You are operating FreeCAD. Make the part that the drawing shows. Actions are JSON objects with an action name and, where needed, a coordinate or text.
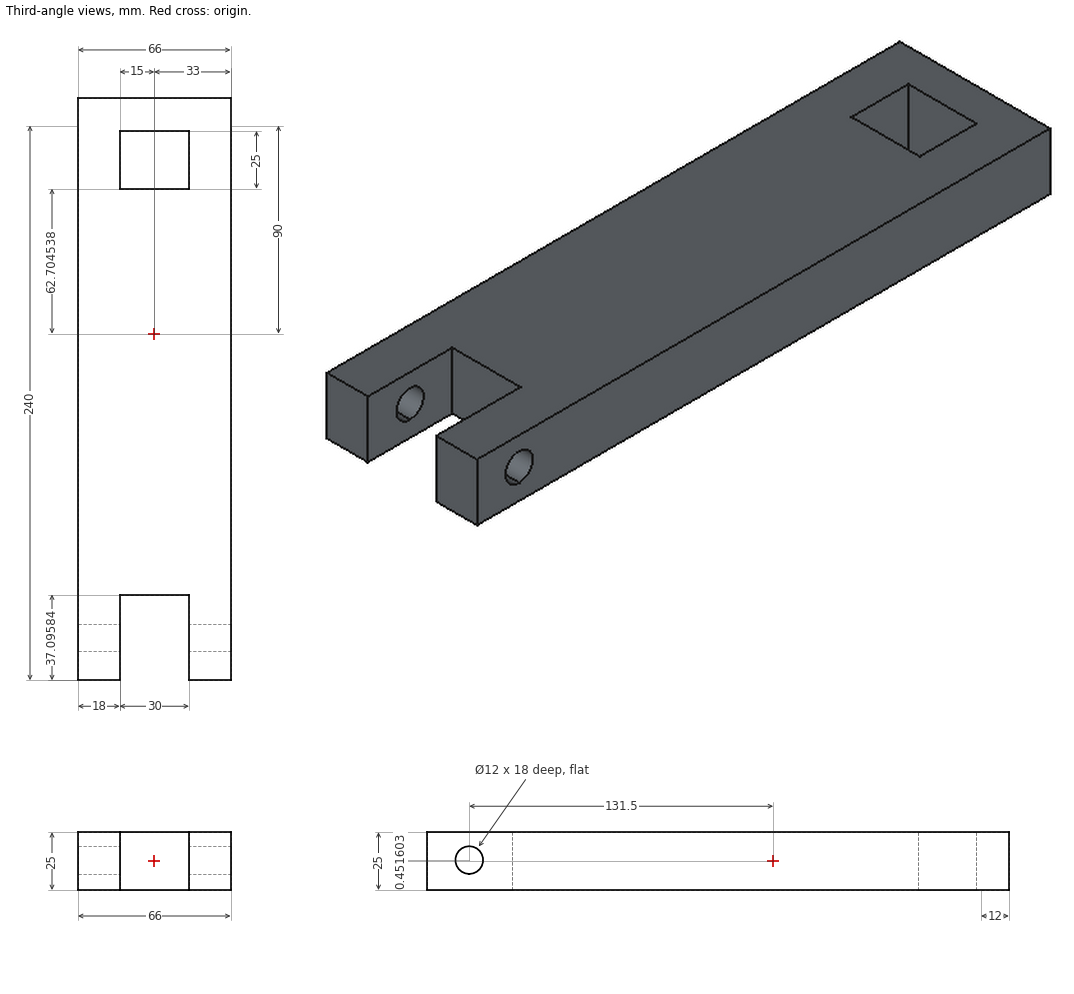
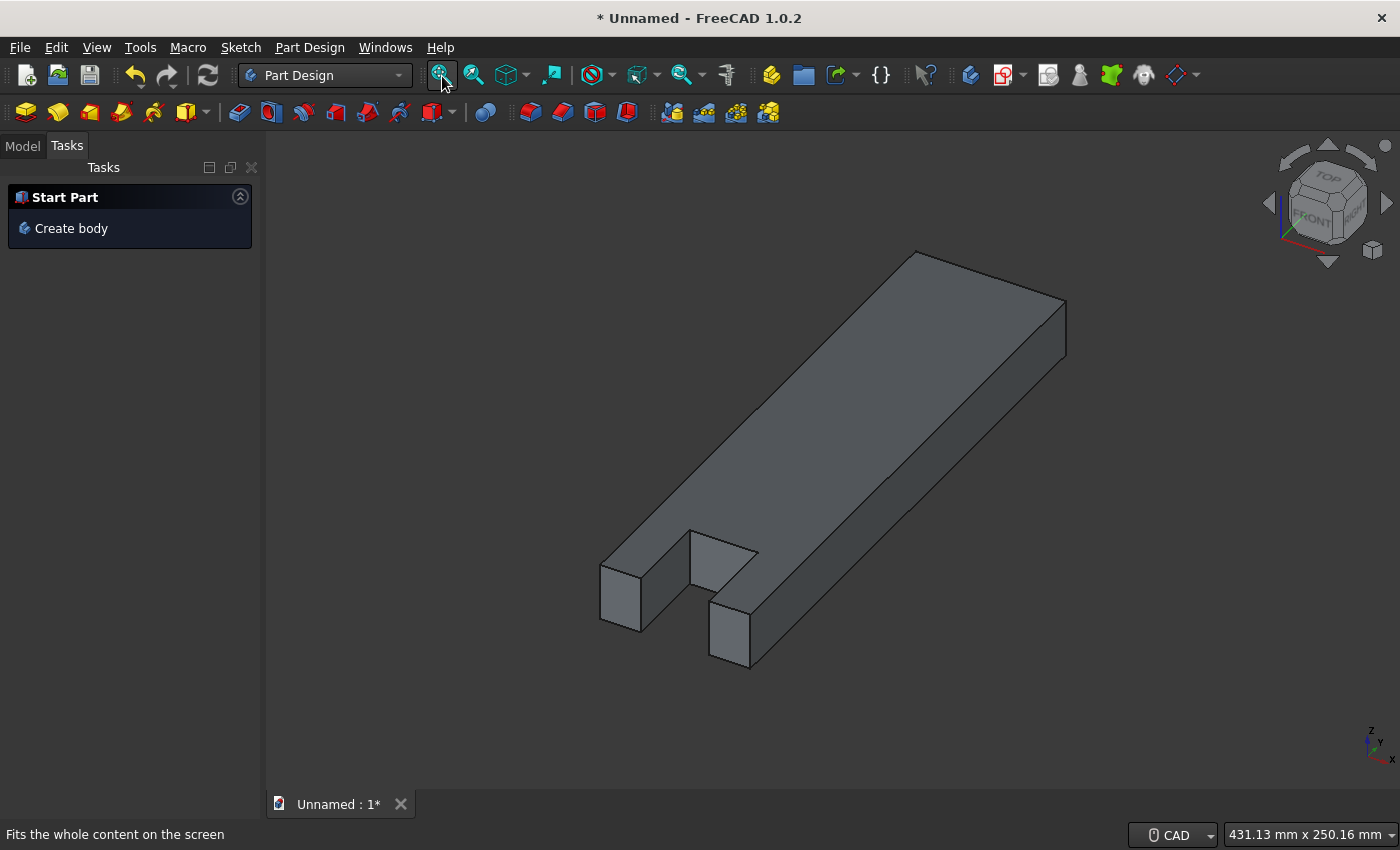
{"action": "left_click", "coordinate": [1043, 350]}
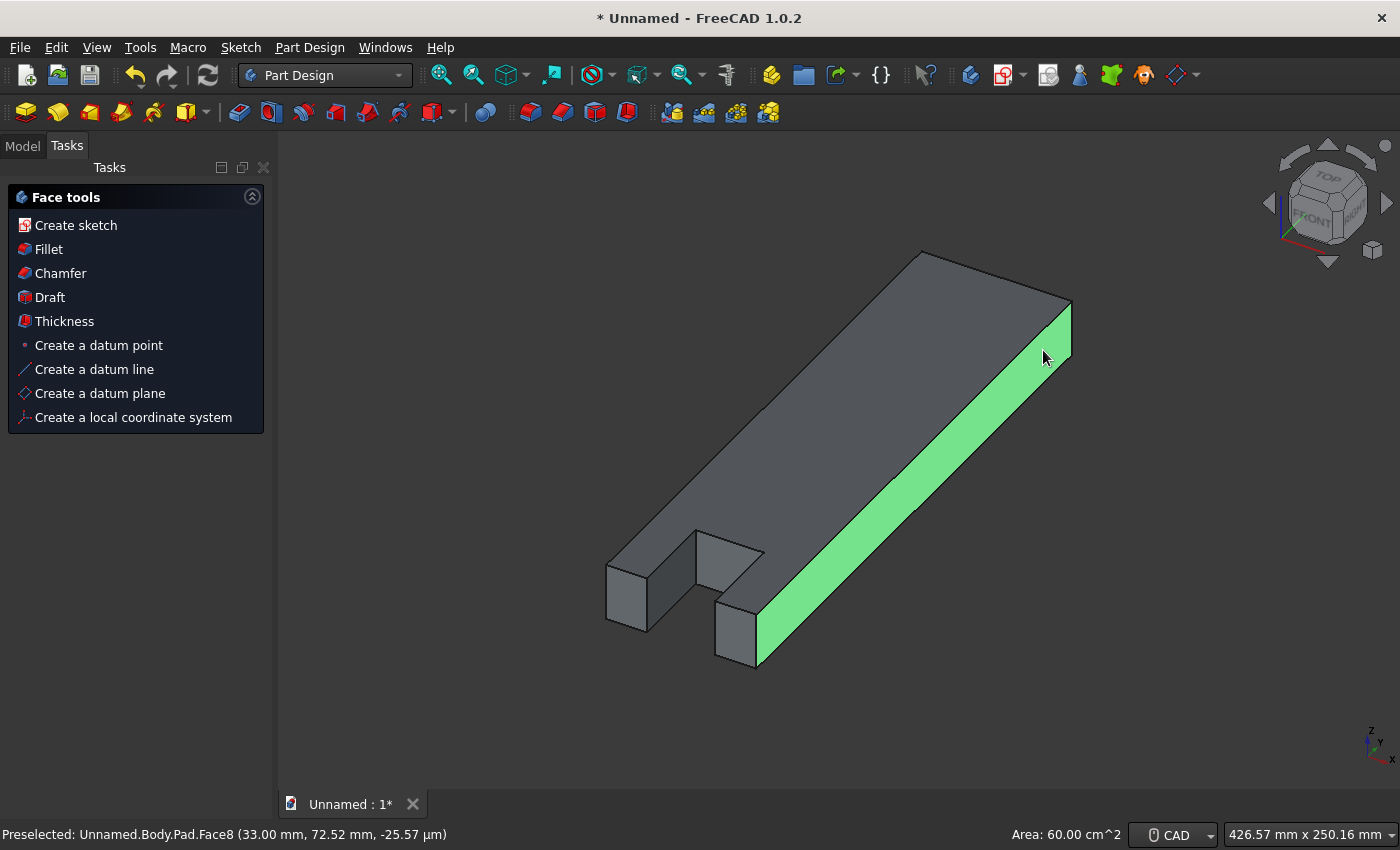
{"action": "left_click", "coordinate": [1004, 76]}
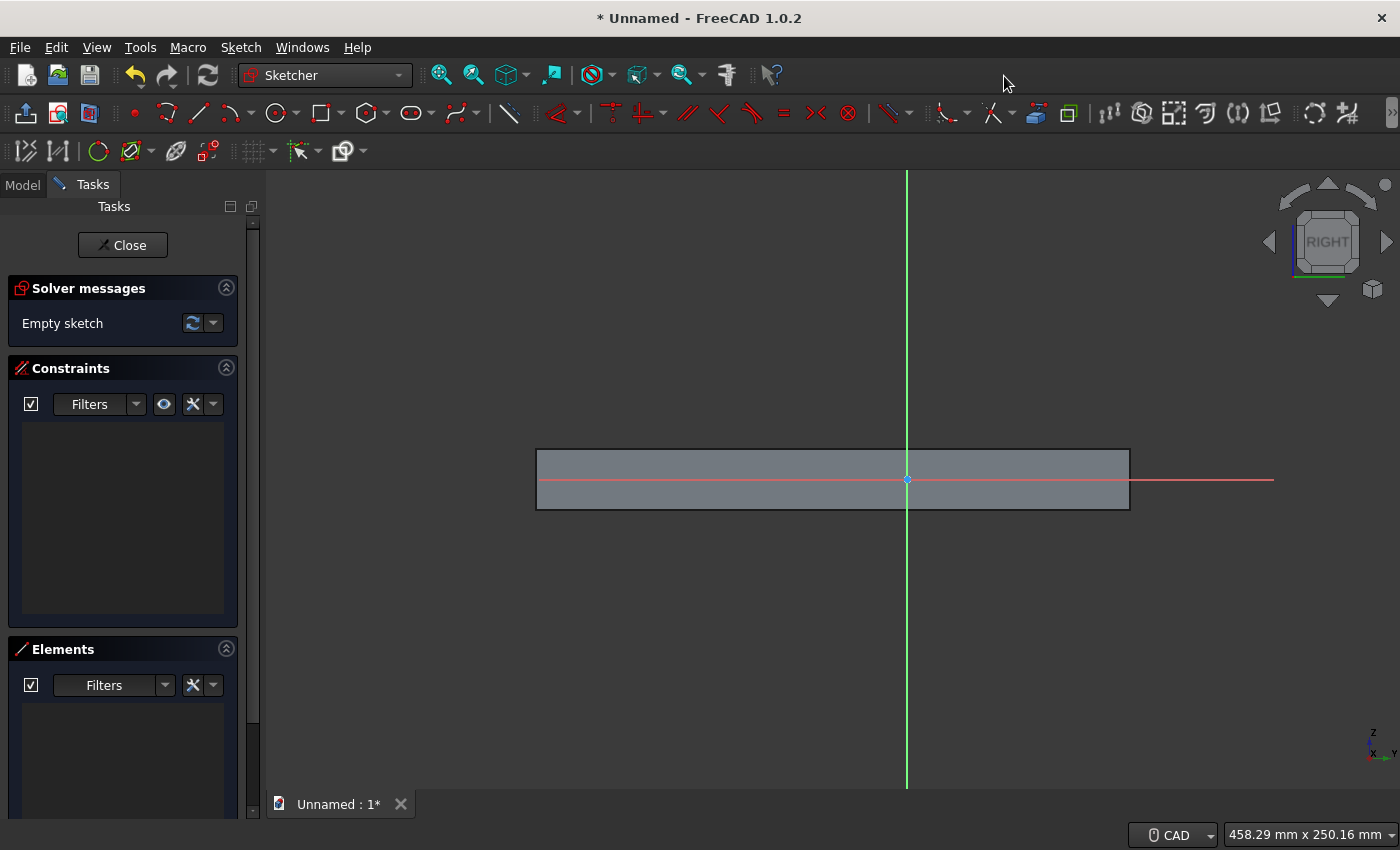
{"action": "scroll", "coordinate": [567, 478], "scroll_direction": "up", "scroll_amount": 13}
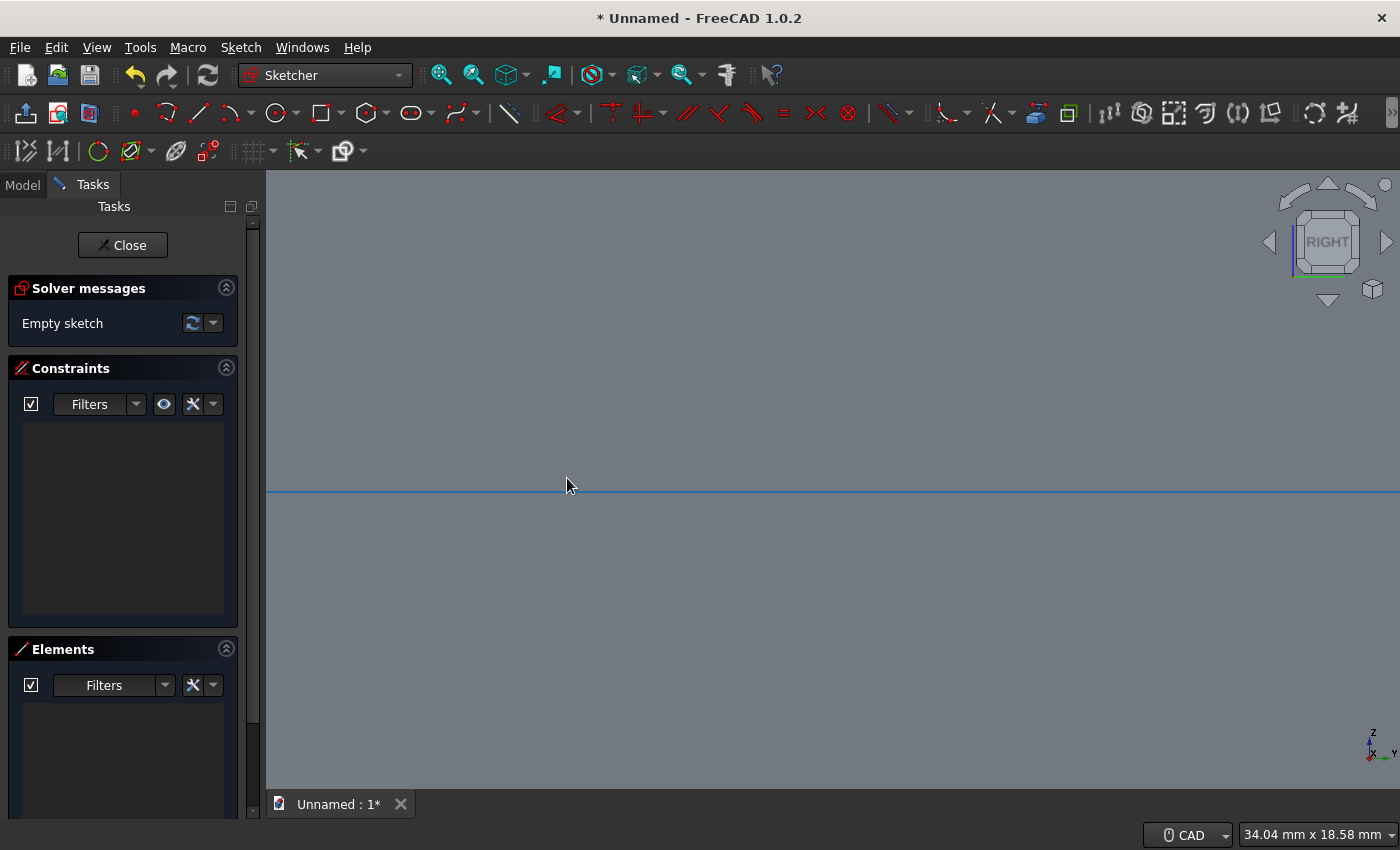
{"action": "left_click", "coordinate": [276, 114]}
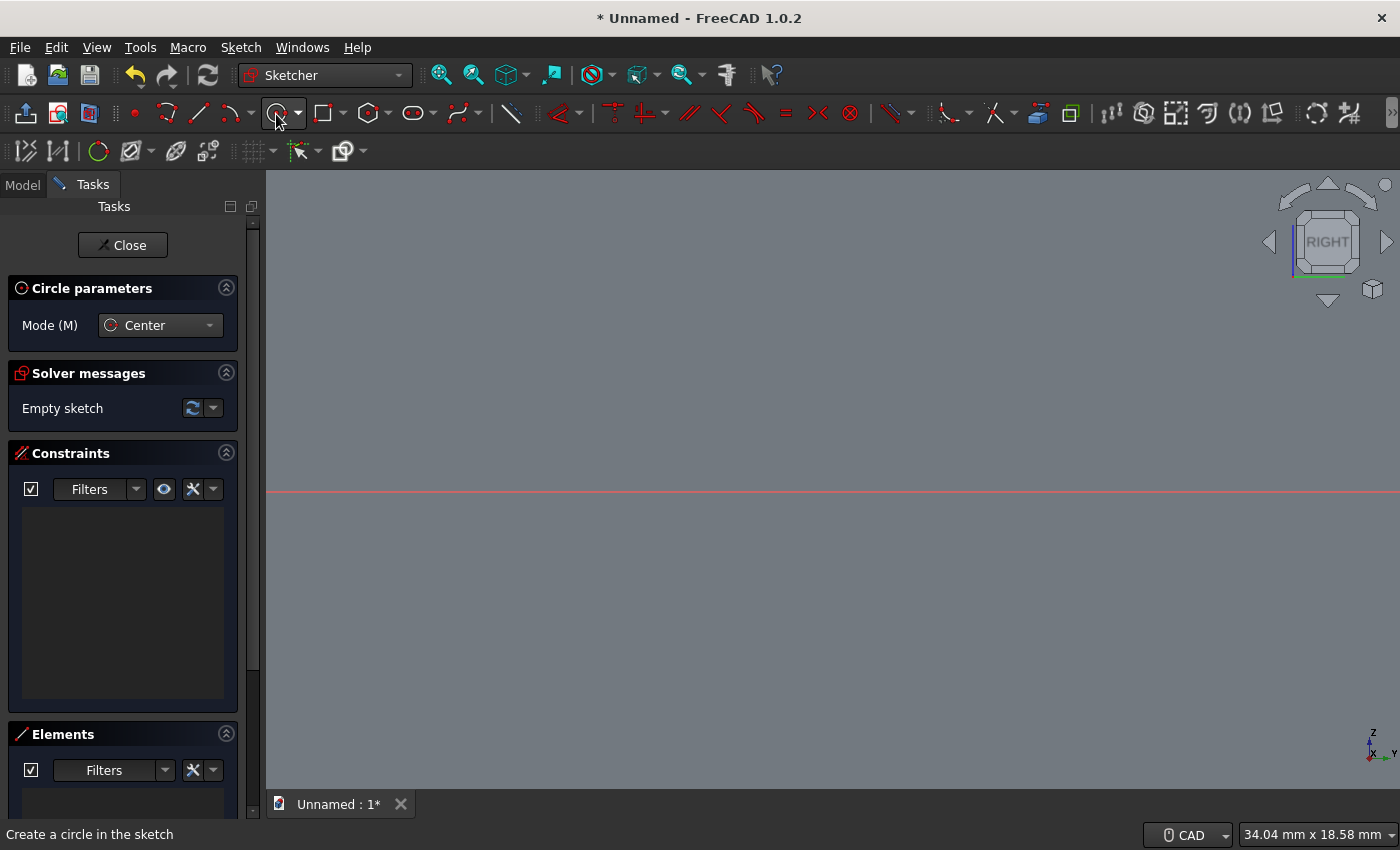
{"action": "left_click", "coordinate": [764, 477]}
{"action": "mouse_move", "coordinate": [905, 336]}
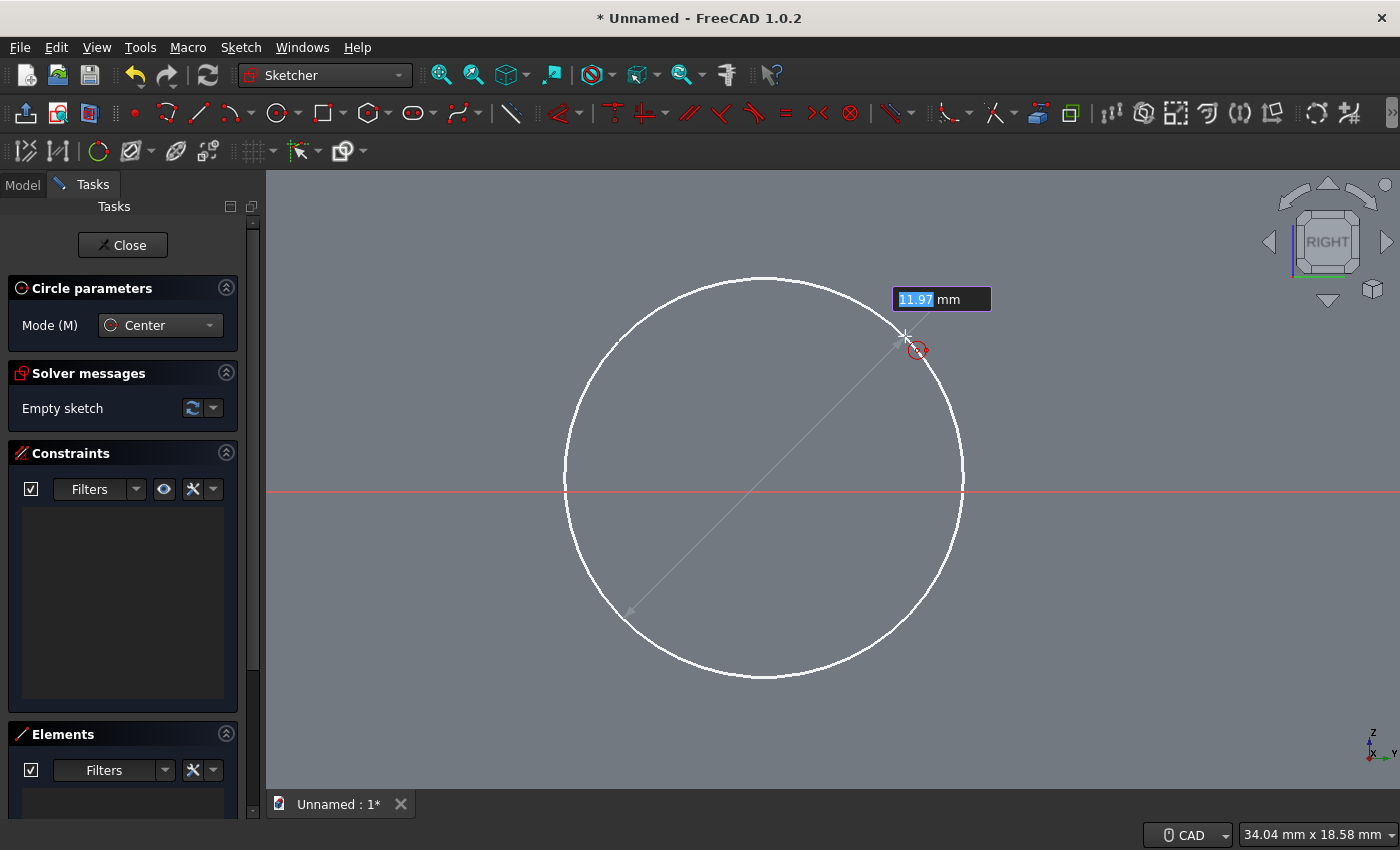
{"action": "type", "text": "12"}
{"action": "key", "text": "Return"}
{"action": "key", "text": "Escape"}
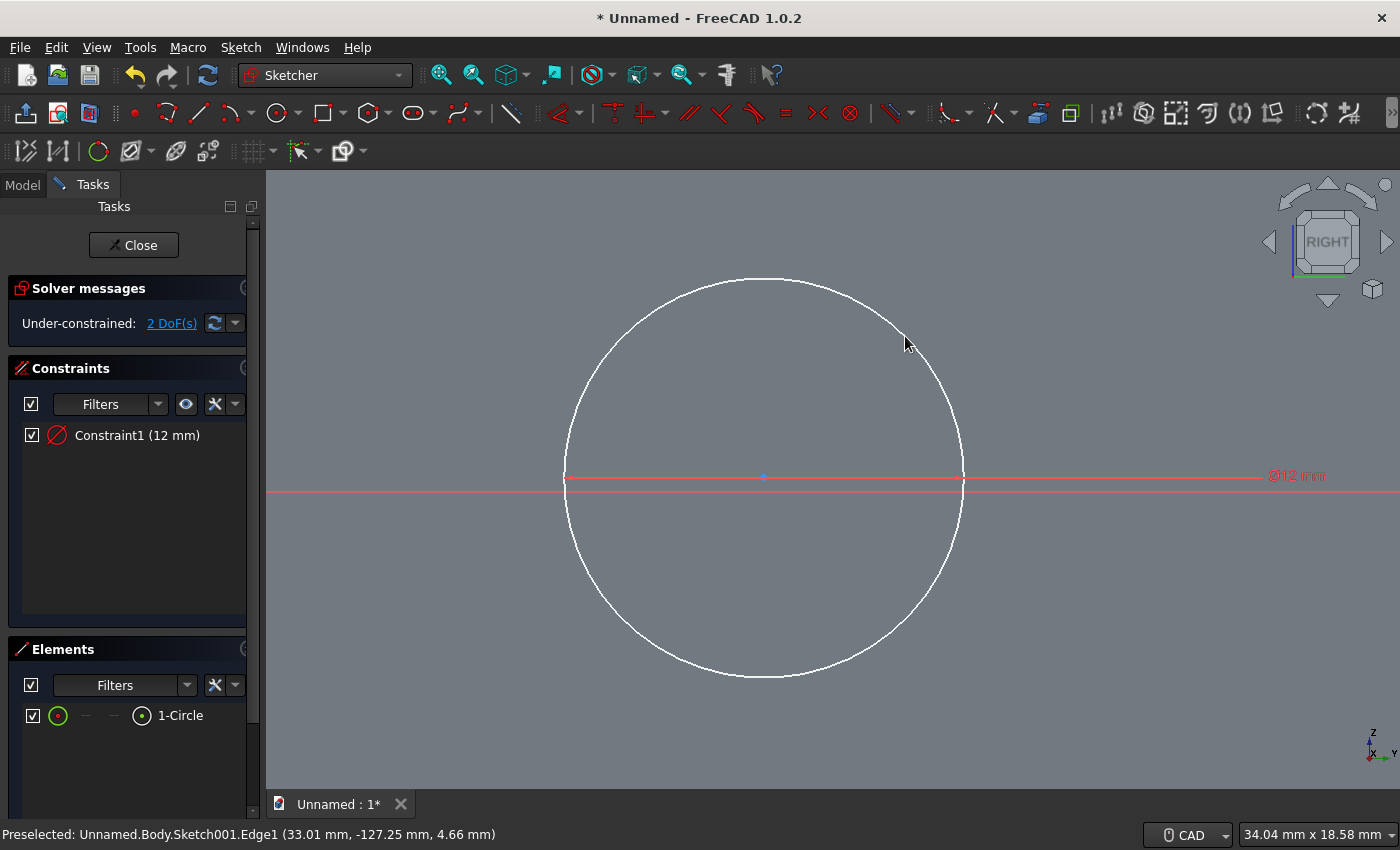
{"action": "left_click", "coordinate": [558, 114]}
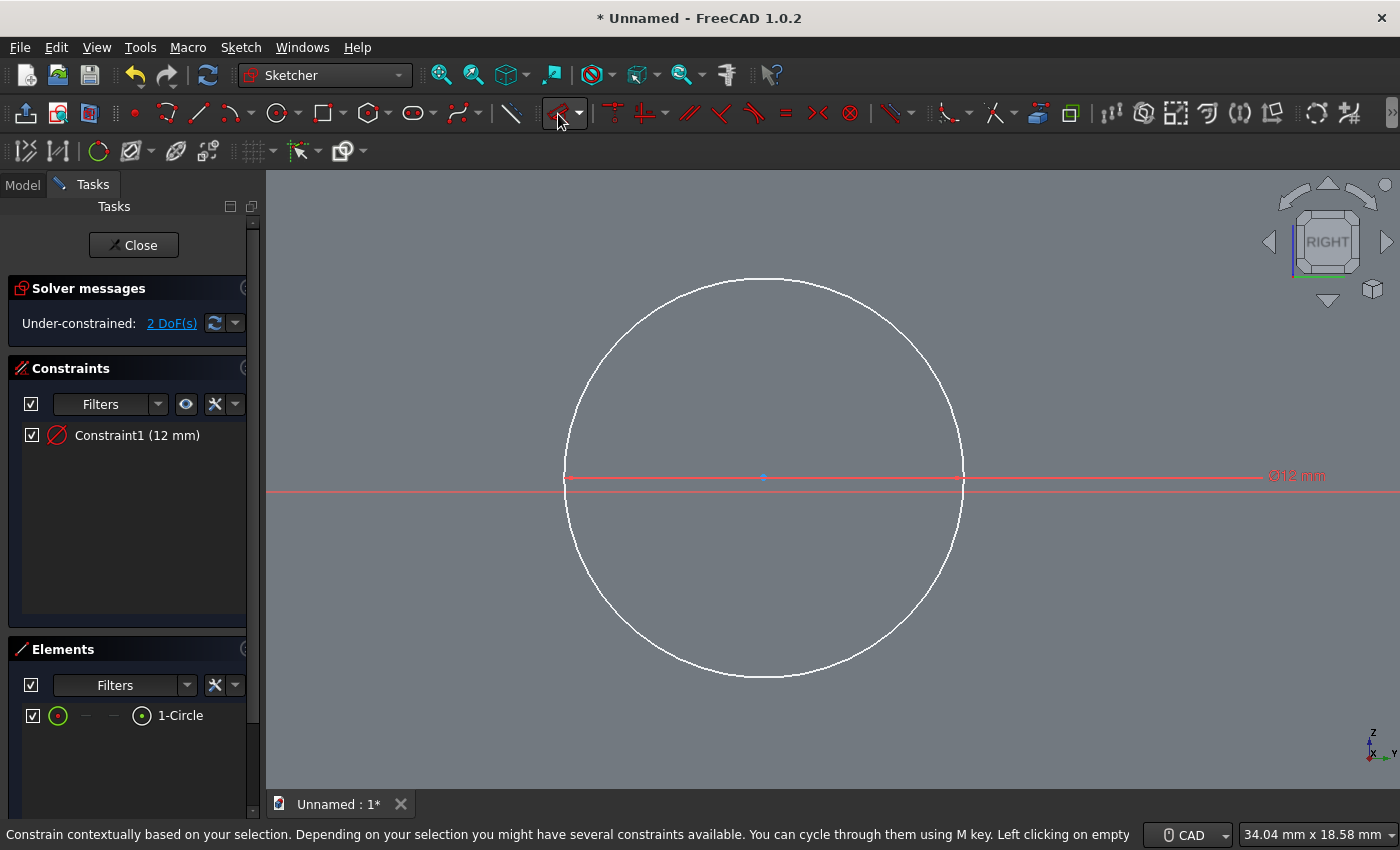
{"action": "left_click", "coordinate": [764, 478]}
{"action": "left_click", "coordinate": [999, 526]}